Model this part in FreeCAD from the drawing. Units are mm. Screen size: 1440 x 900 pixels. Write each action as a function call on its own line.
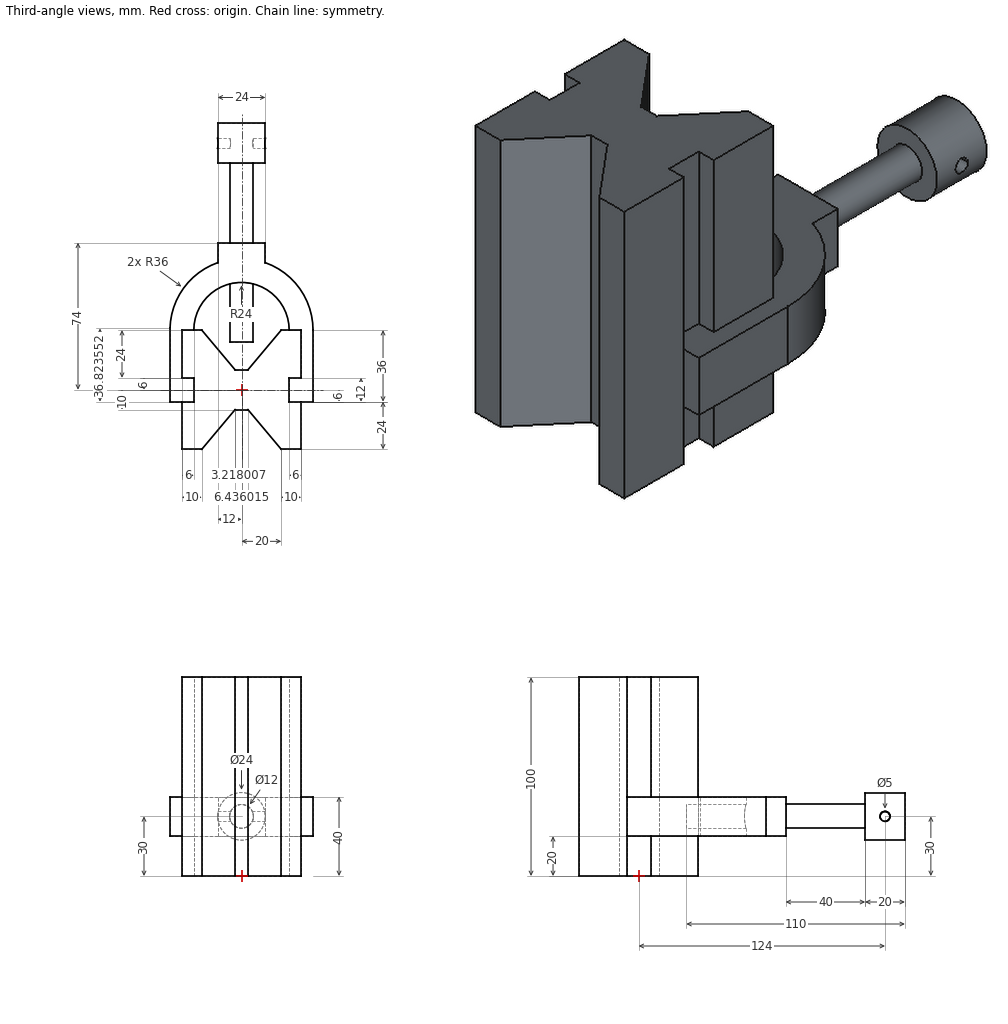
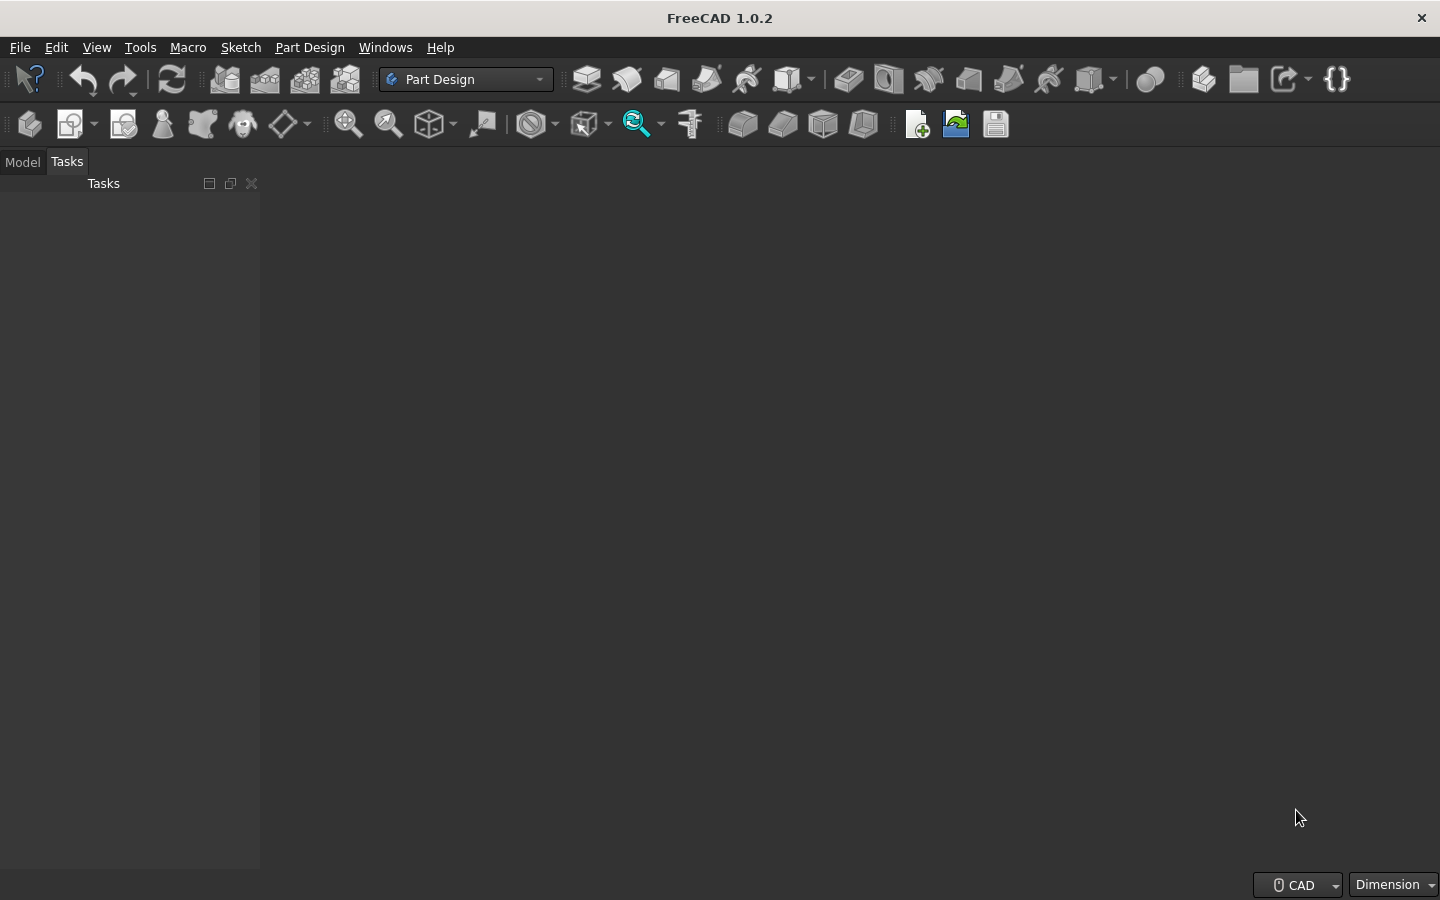
key(ctrl+n)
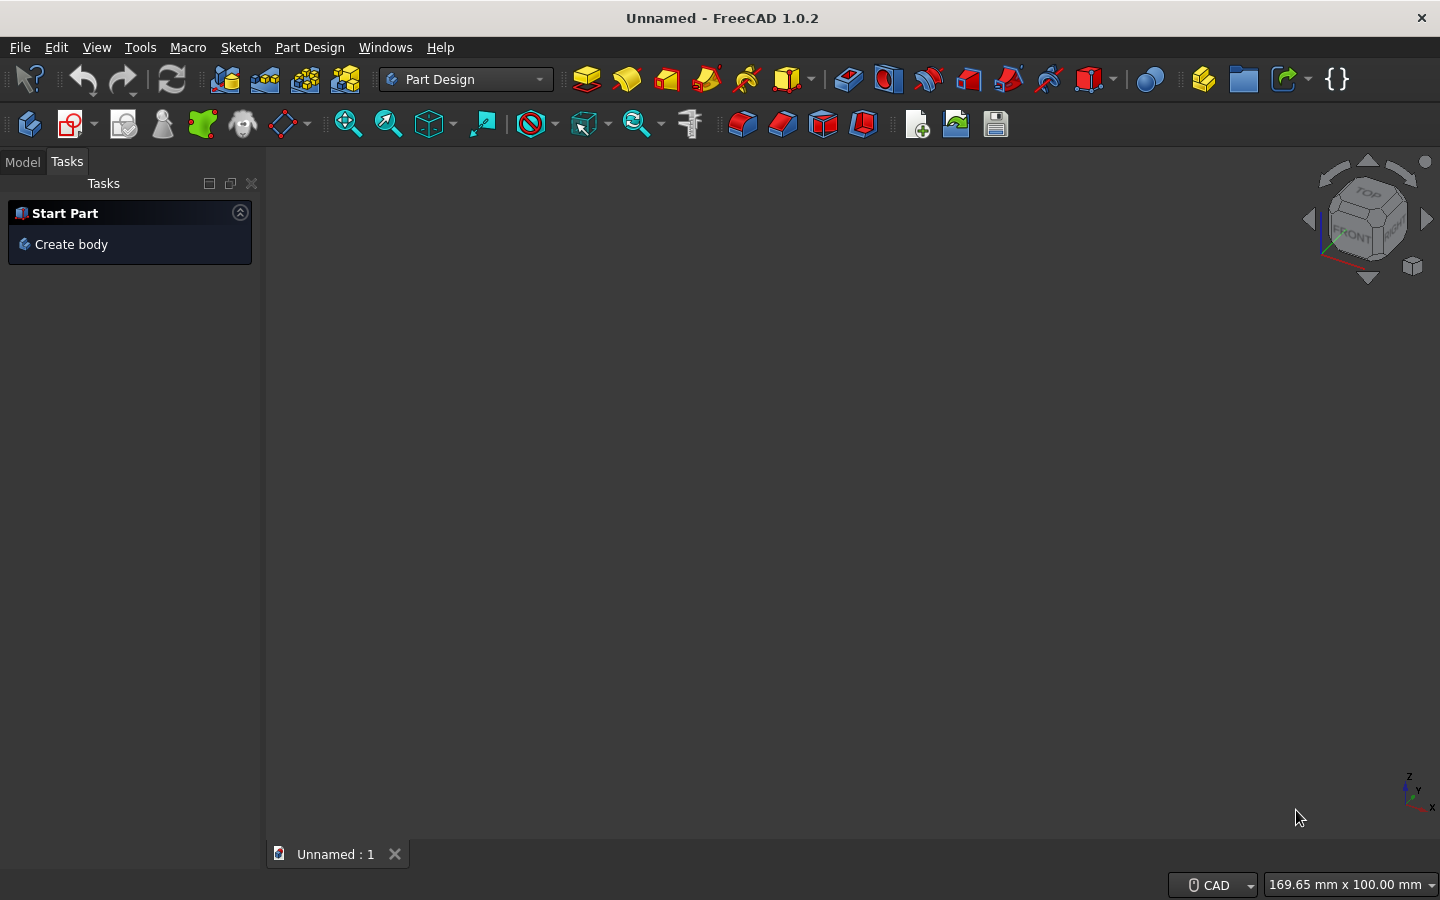
click(70, 124)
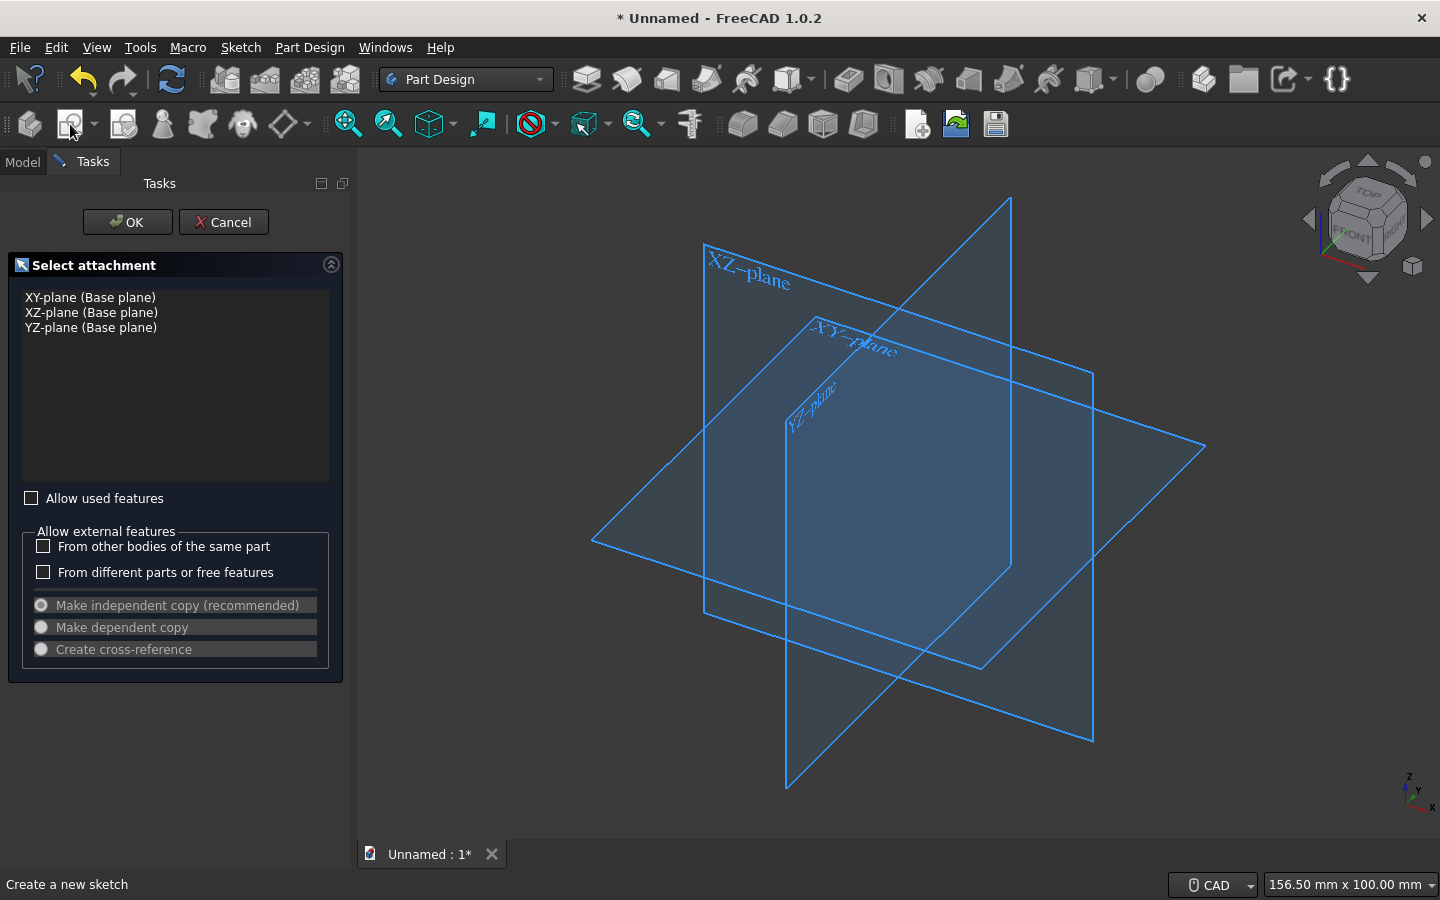
click(82, 298)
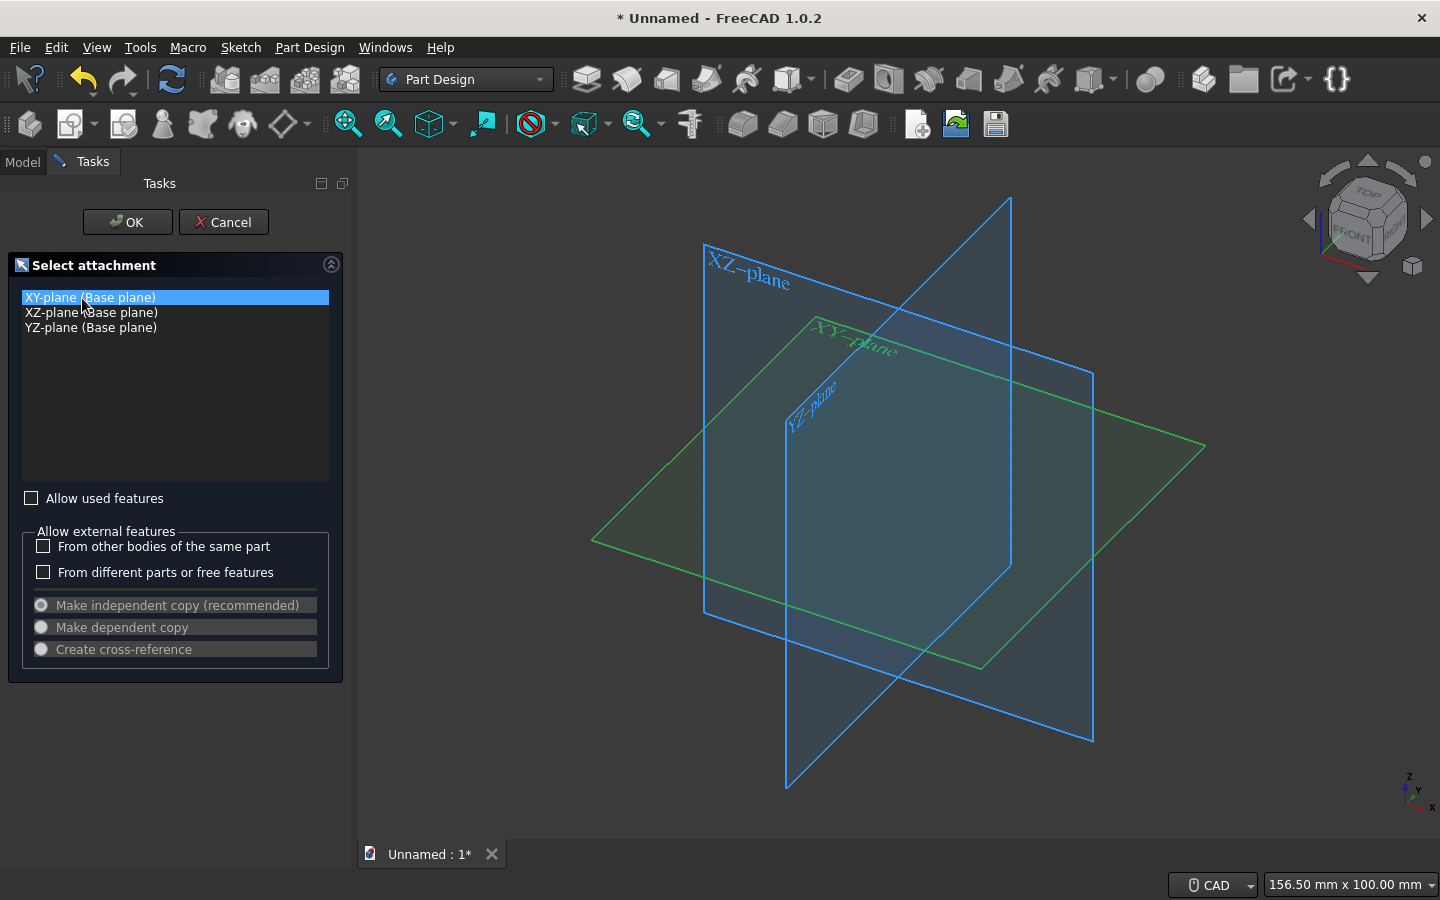
click(128, 222)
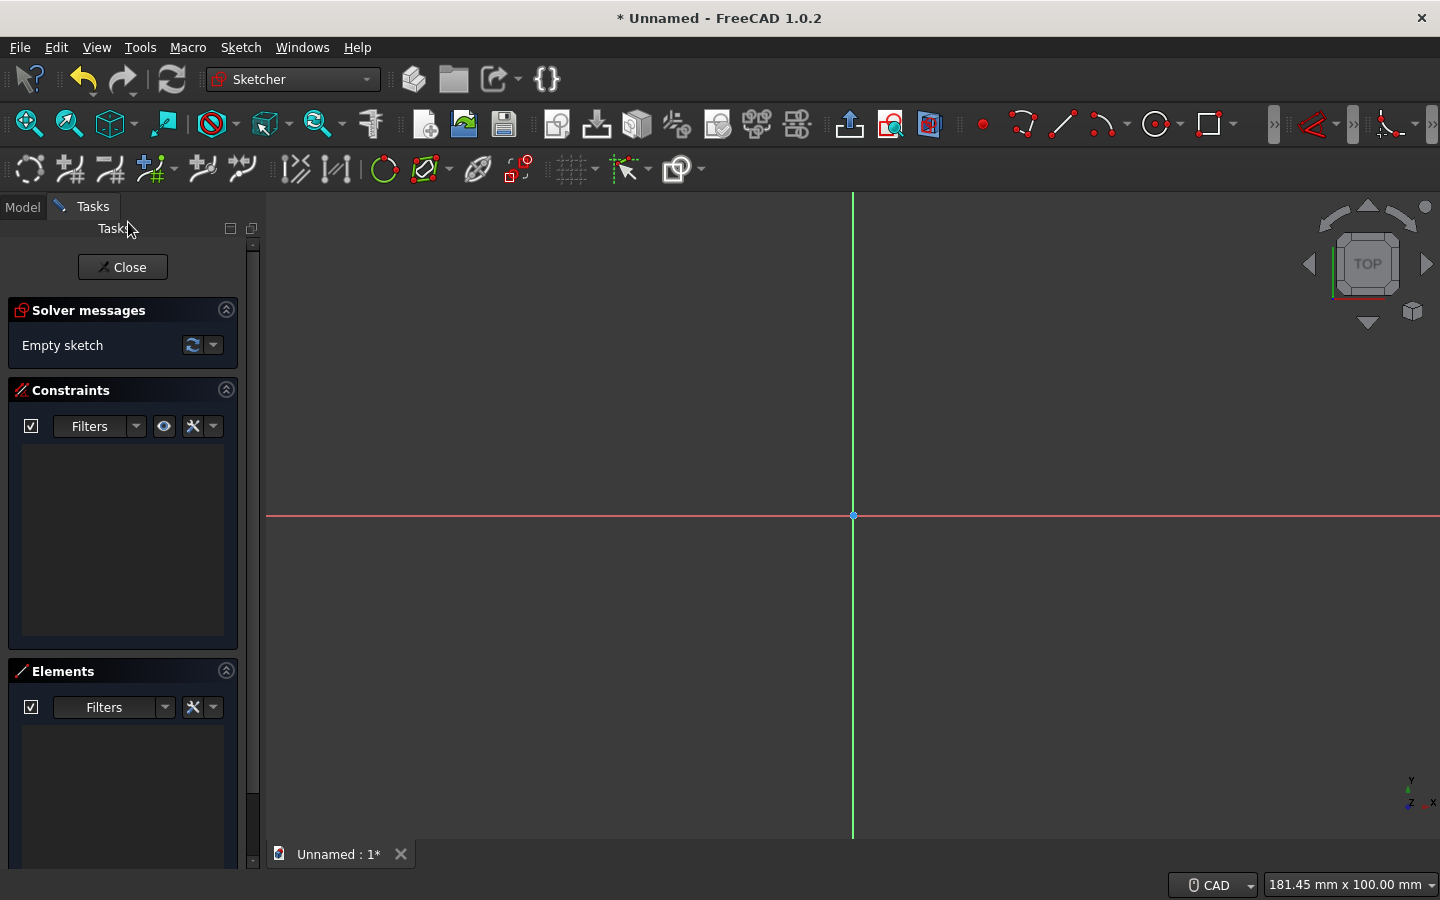
key(g)
key(m)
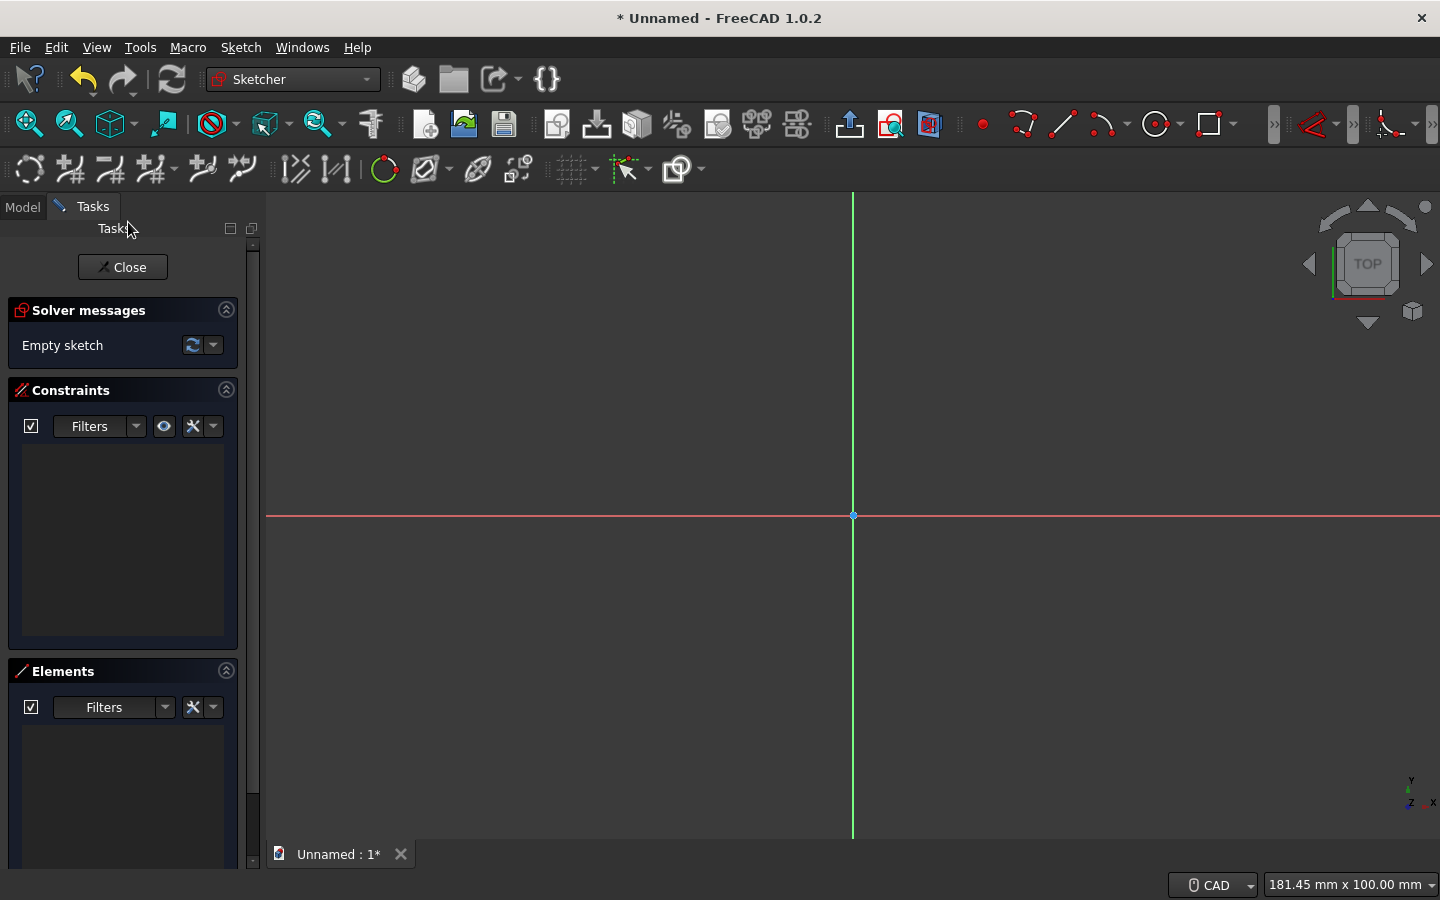
click(832, 580)
click(874, 580)
click(982, 710)
click(1047, 710)
click(1047, 554)
click(1008, 554)
click(1008, 477)
click(1047, 477)
click(1047, 321)
click(982, 321)
click(874, 451)
click(832, 451)
click(724, 321)
click(659, 321)
click(659, 477)
click(698, 477)
click(698, 554)
click(659, 554)
click(659, 710)
click(724, 710)
click(832, 581)
key(Escape)
key(Escape)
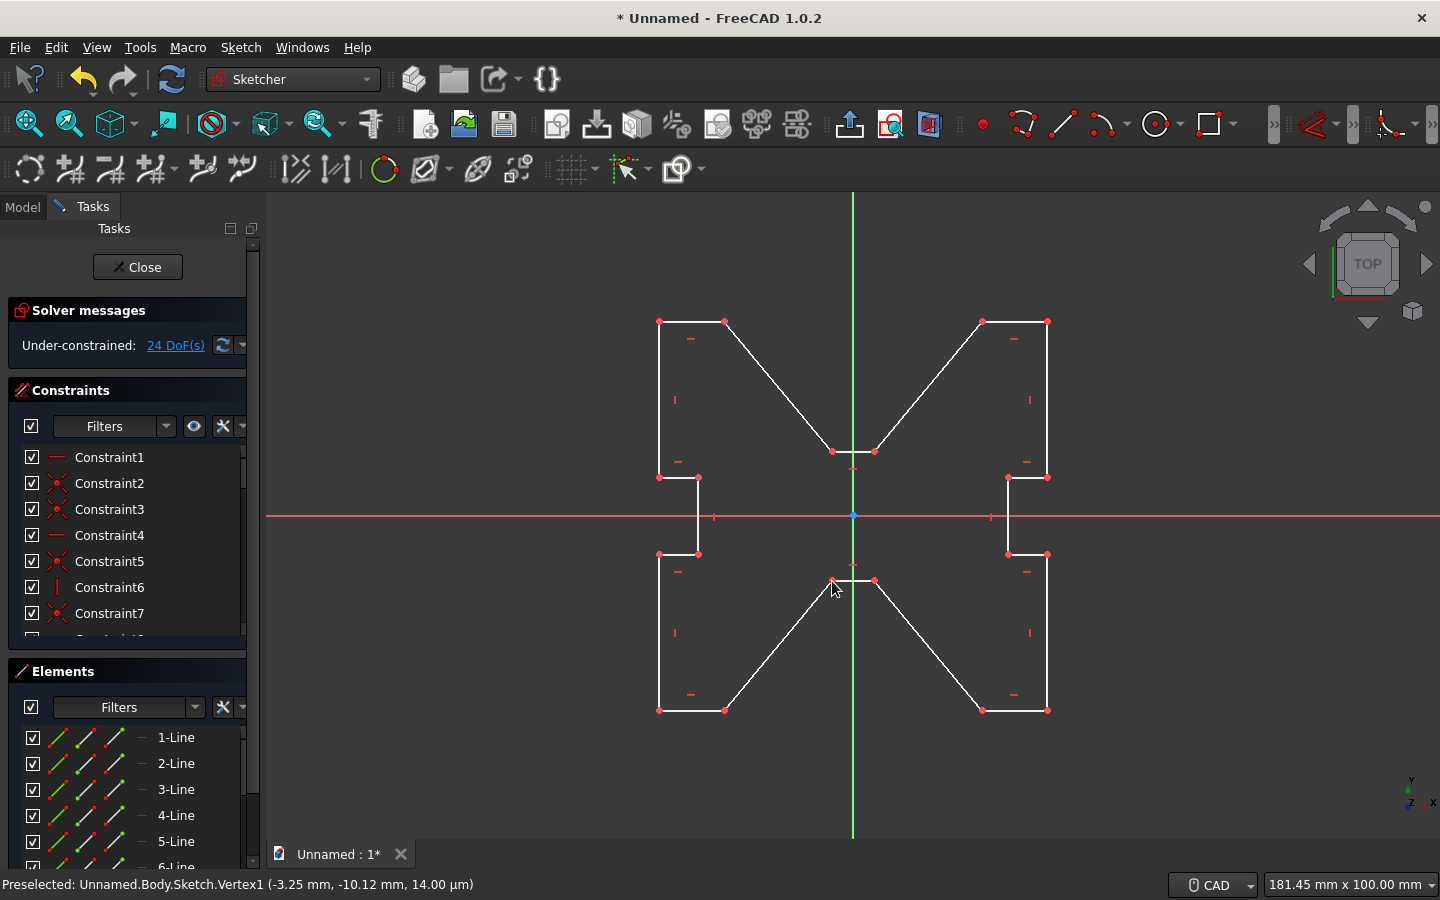
click(1047, 555)